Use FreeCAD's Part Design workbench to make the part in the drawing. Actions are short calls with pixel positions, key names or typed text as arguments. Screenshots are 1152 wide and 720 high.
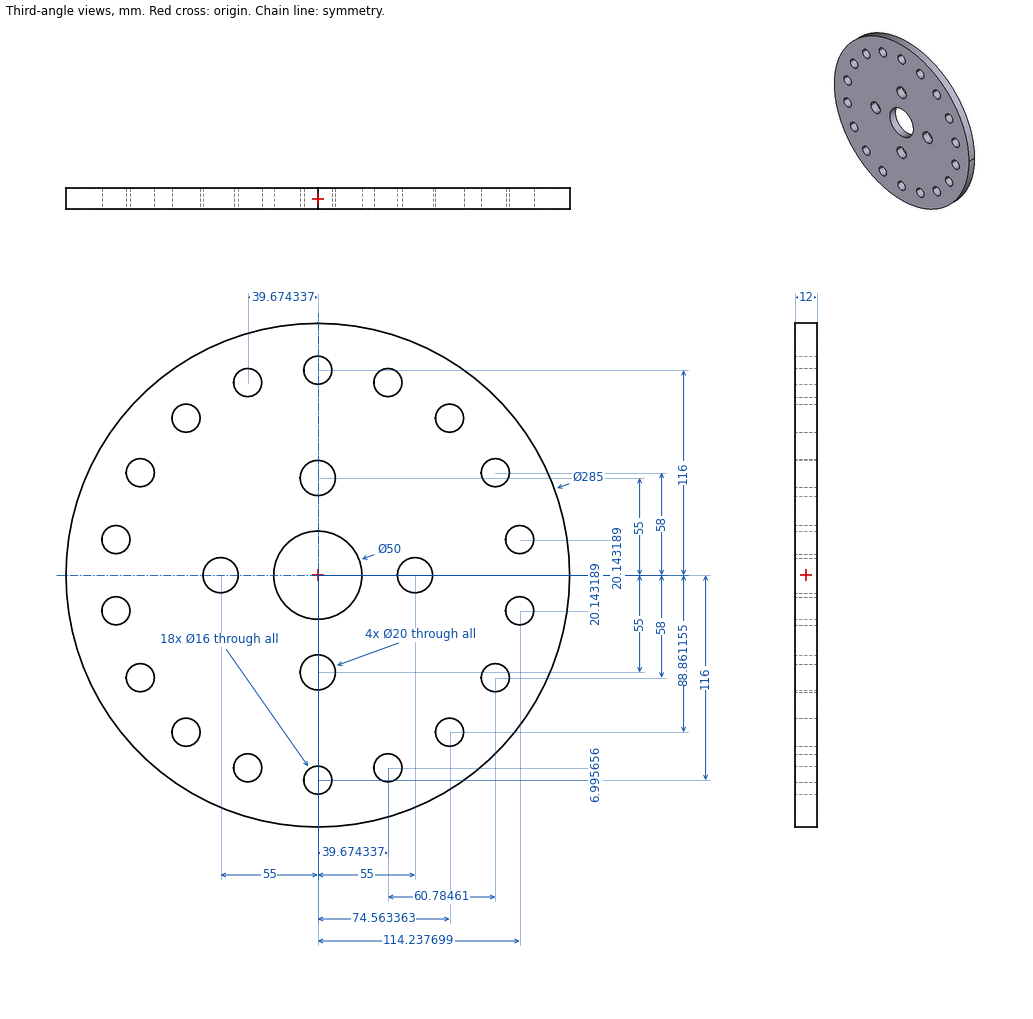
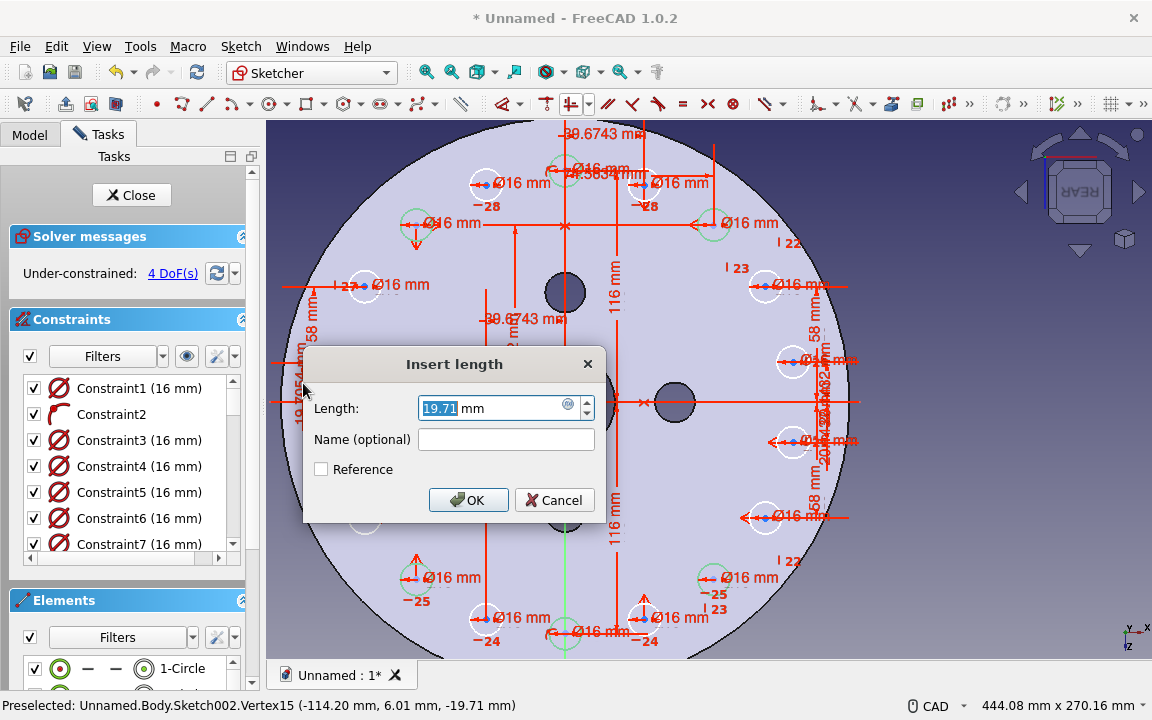
text(20.143189)
key(Return)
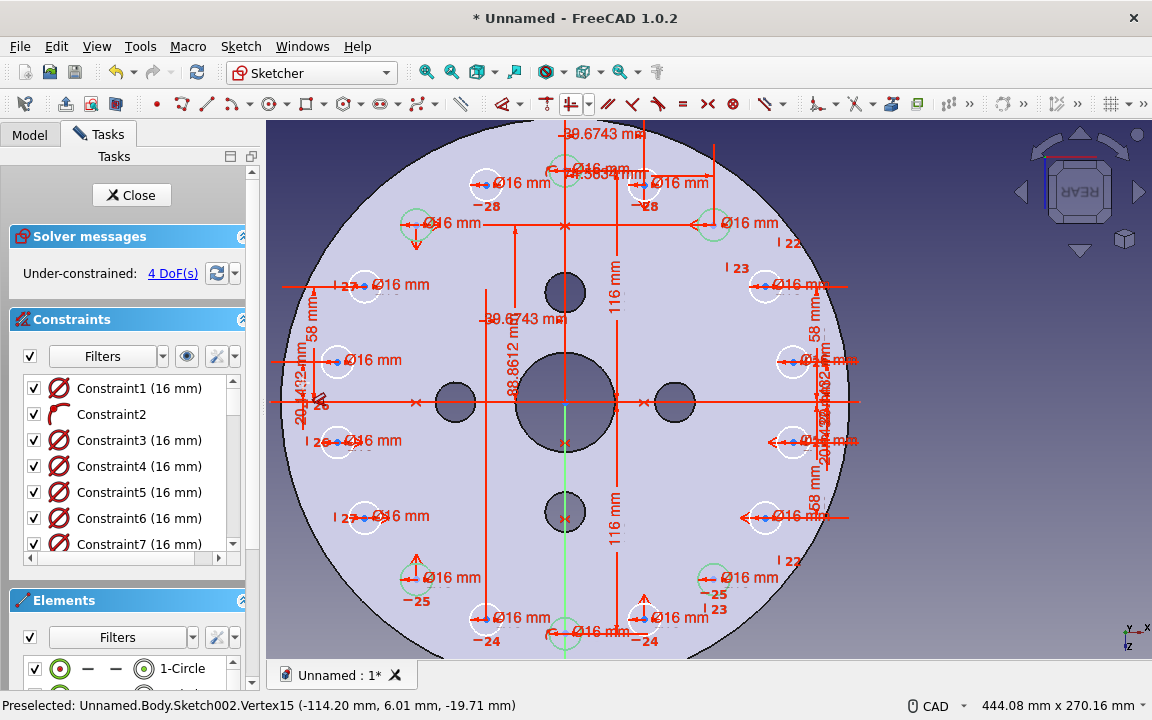
click(486, 185)
click(526, 151)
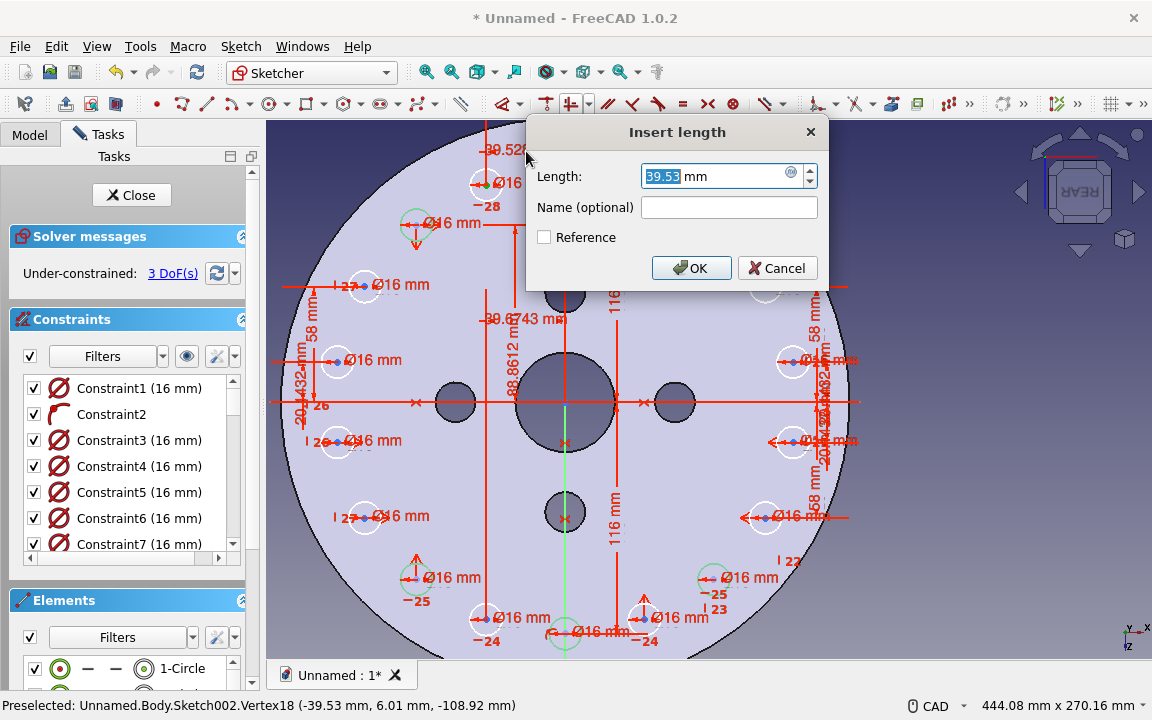
text(39.674337)
key(Return)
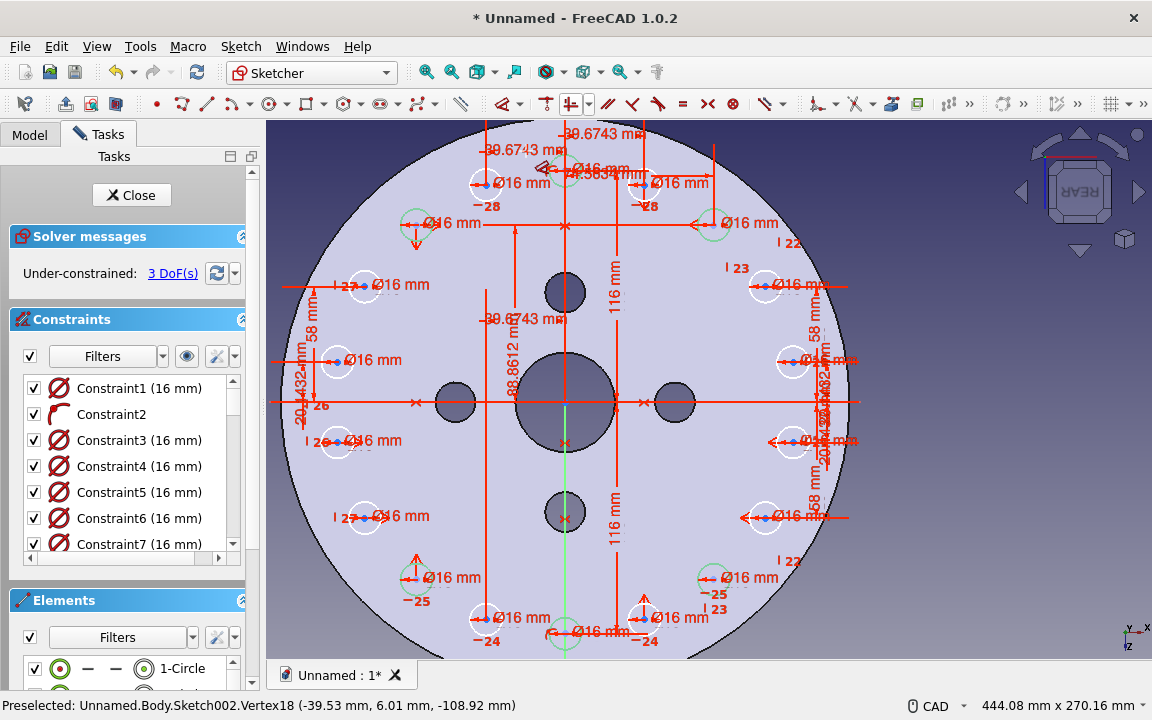
scroll(565, 171, up, 6)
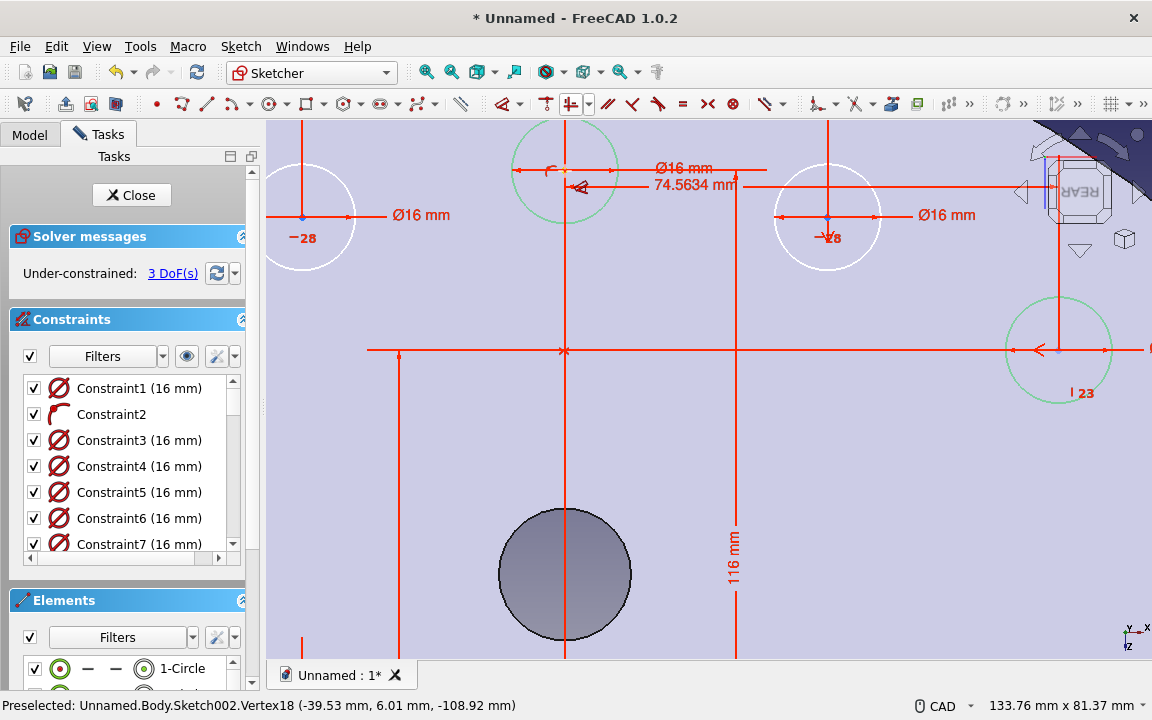
click(565, 170)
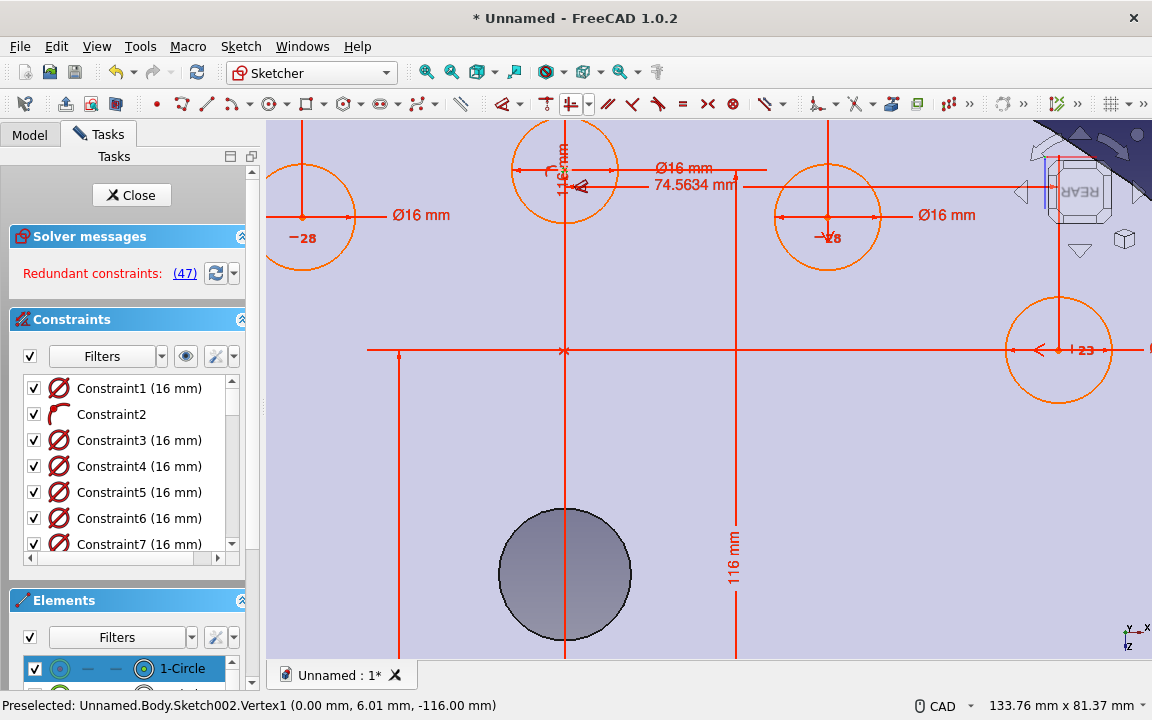
click(828, 217)
click(862, 205)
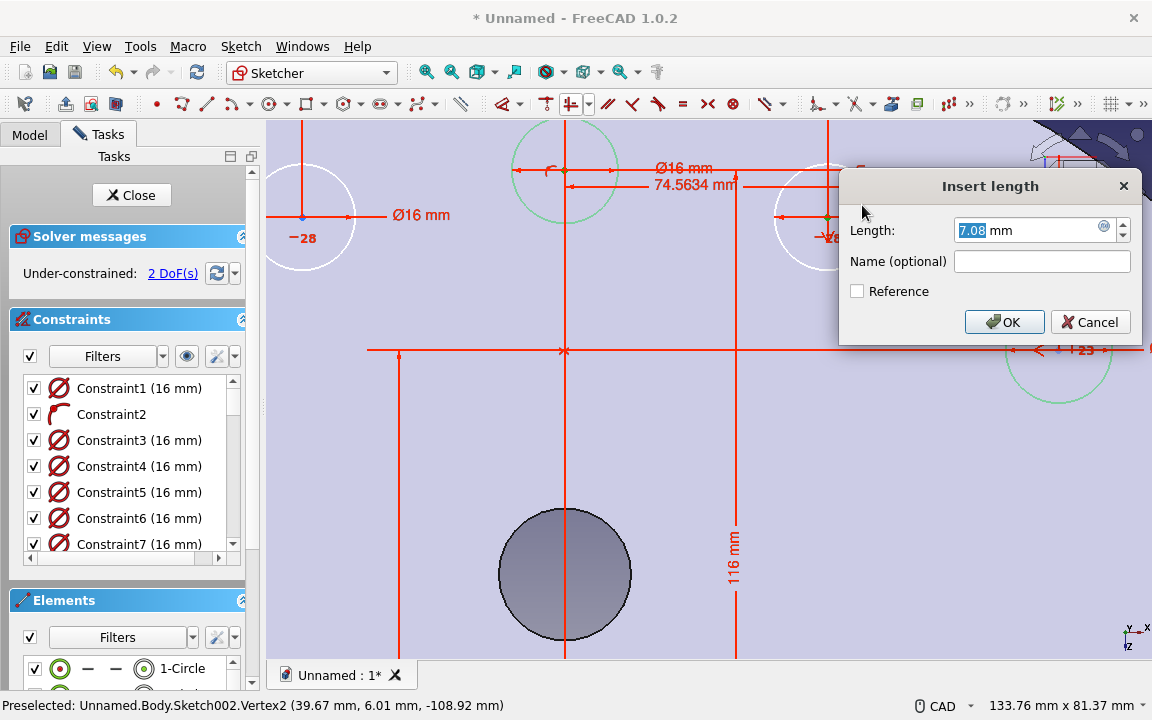
text(6.995656)
key(Return)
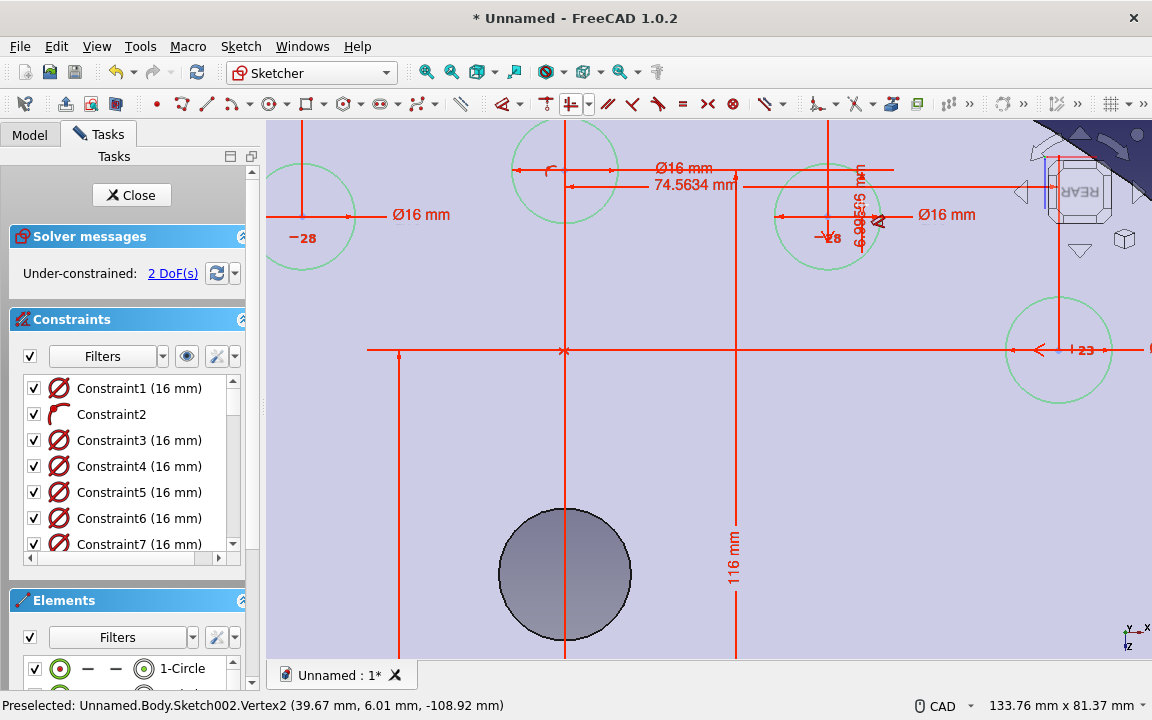
scroll(660, 251, down, 8)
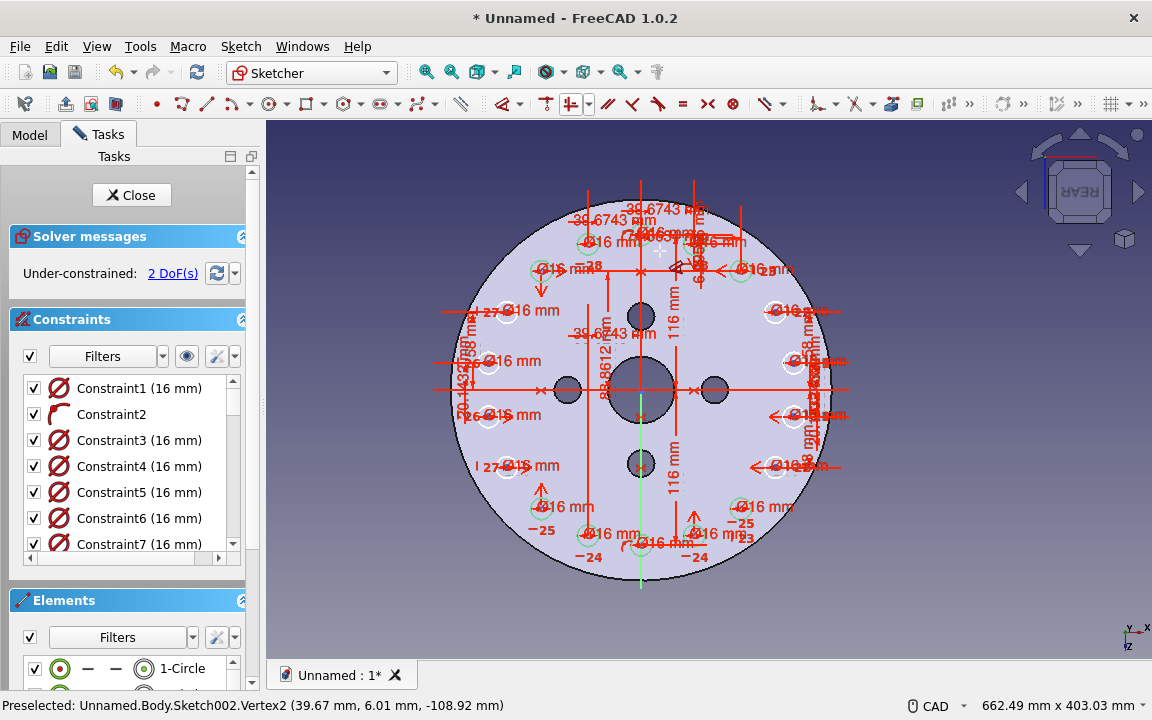
click(694, 244)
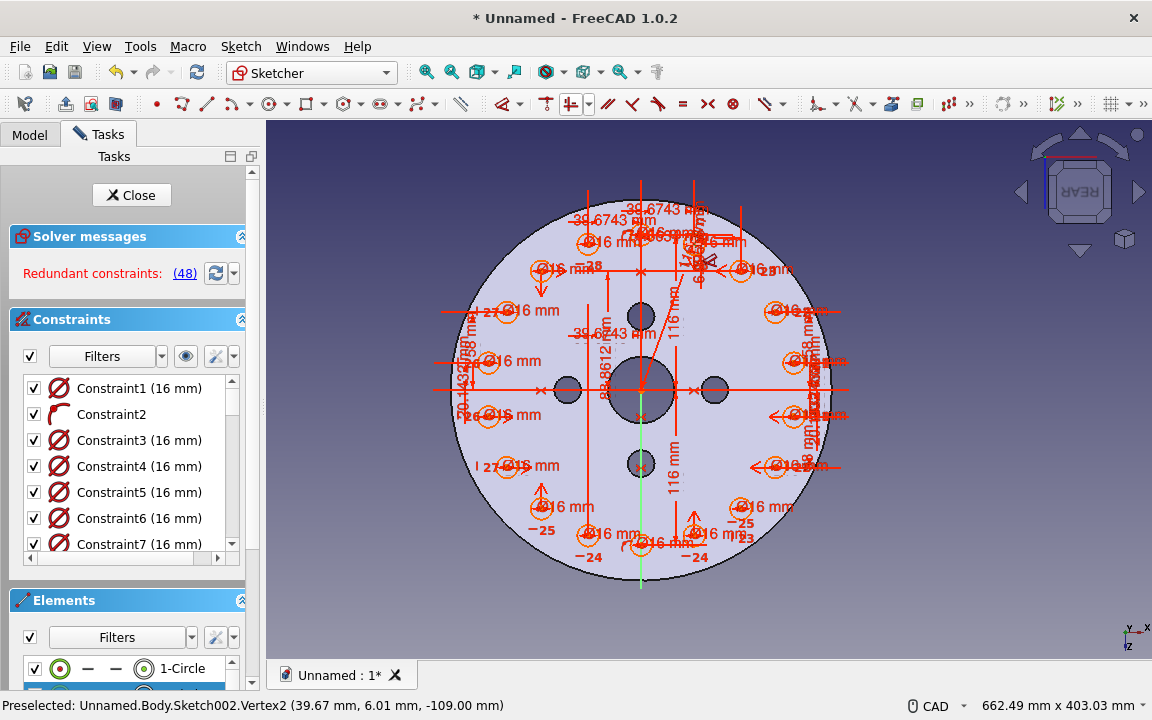
click(775, 312)
click(753, 210)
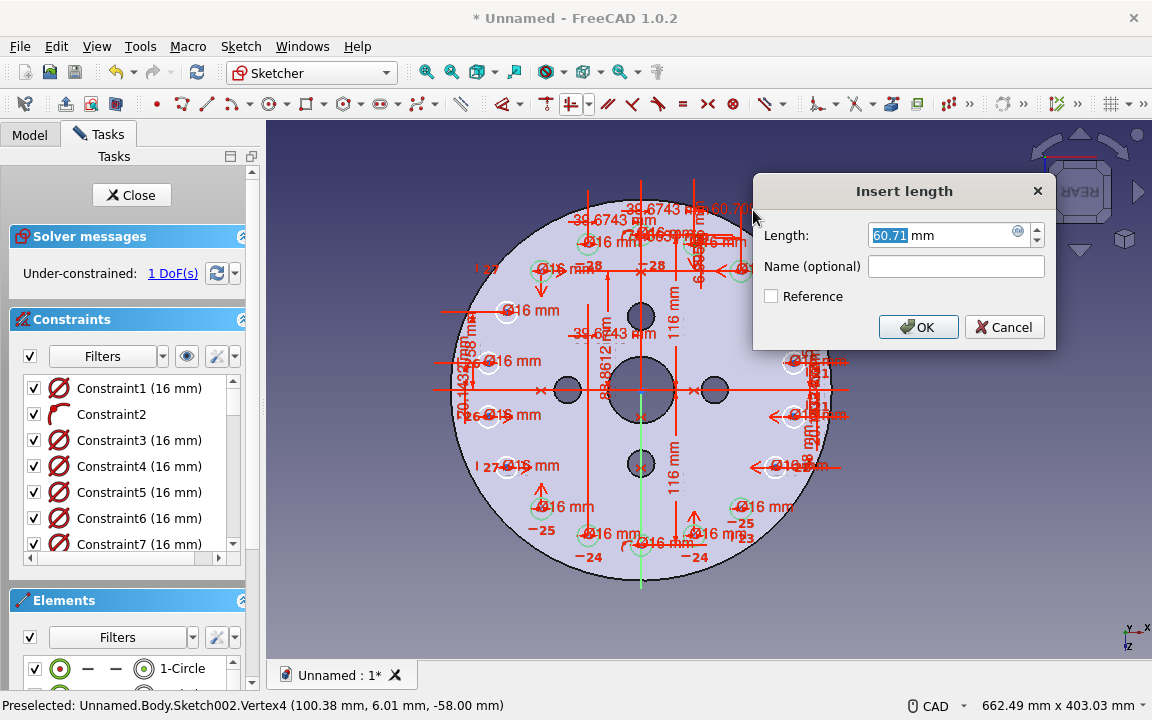
text(60.78461)
key(Return)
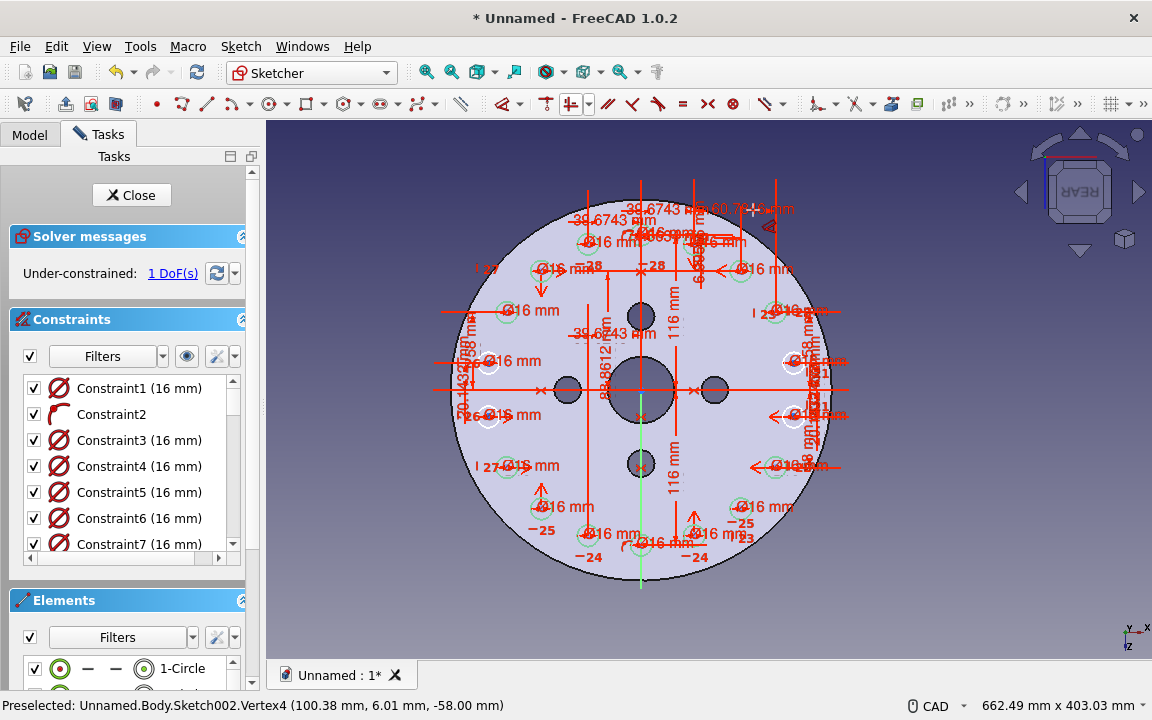
click(794, 363)
click(718, 424)